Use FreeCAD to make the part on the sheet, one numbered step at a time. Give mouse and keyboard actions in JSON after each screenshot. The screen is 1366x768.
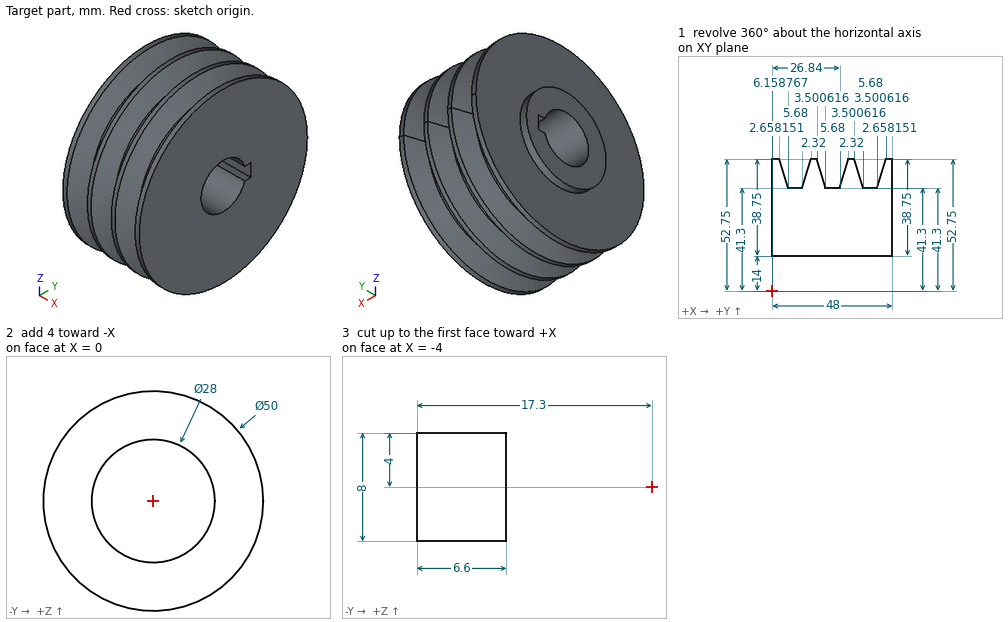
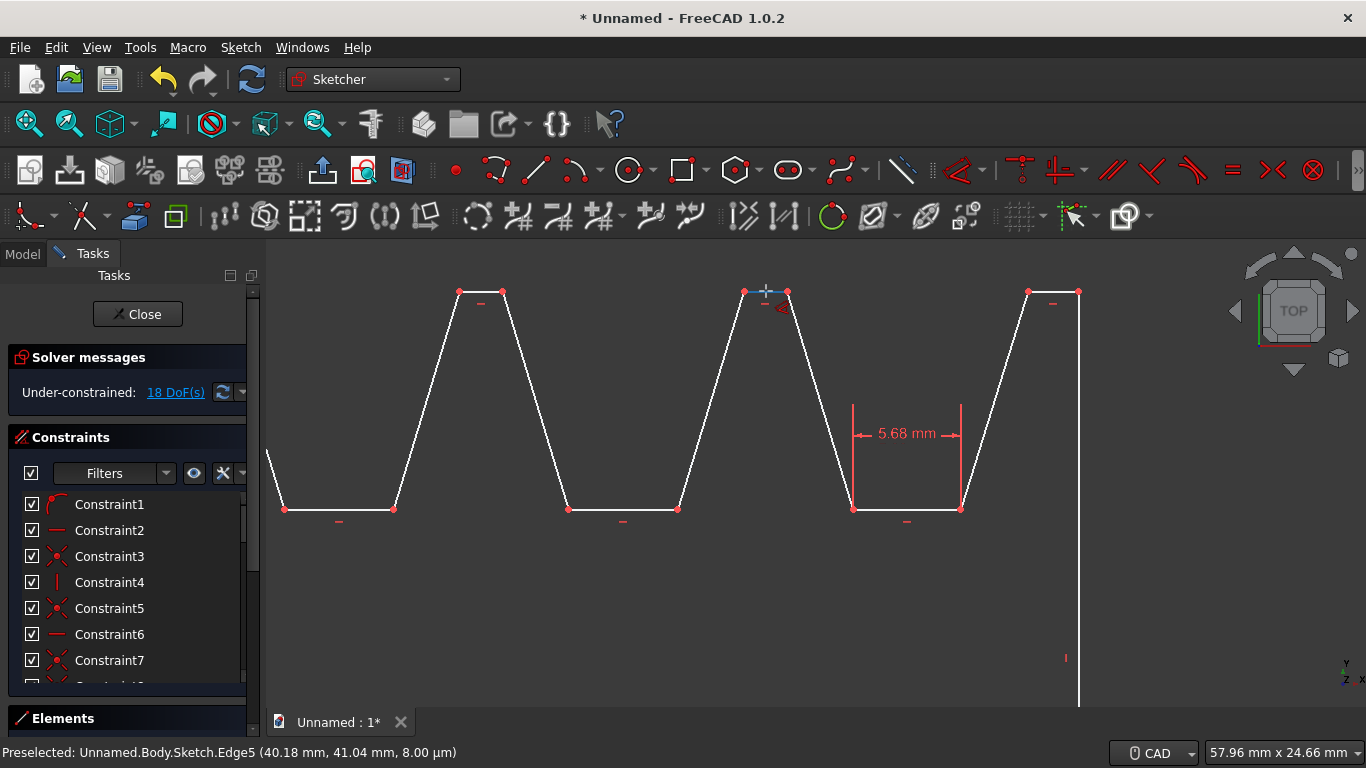
{"action": "left_click", "coordinate": [766, 292]}
{"action": "left_click", "coordinate": [766, 326]}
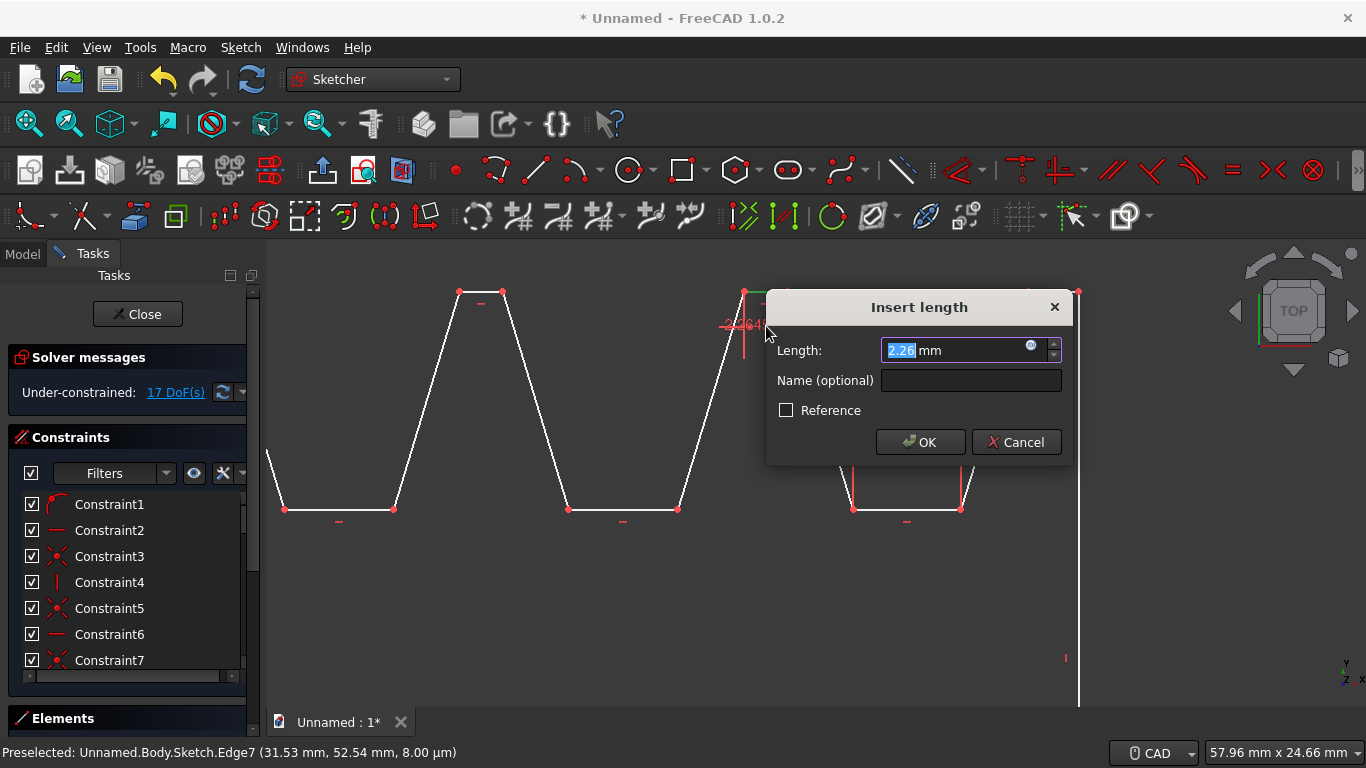
{"action": "type", "text": "2.32"}
{"action": "key", "text": "Return"}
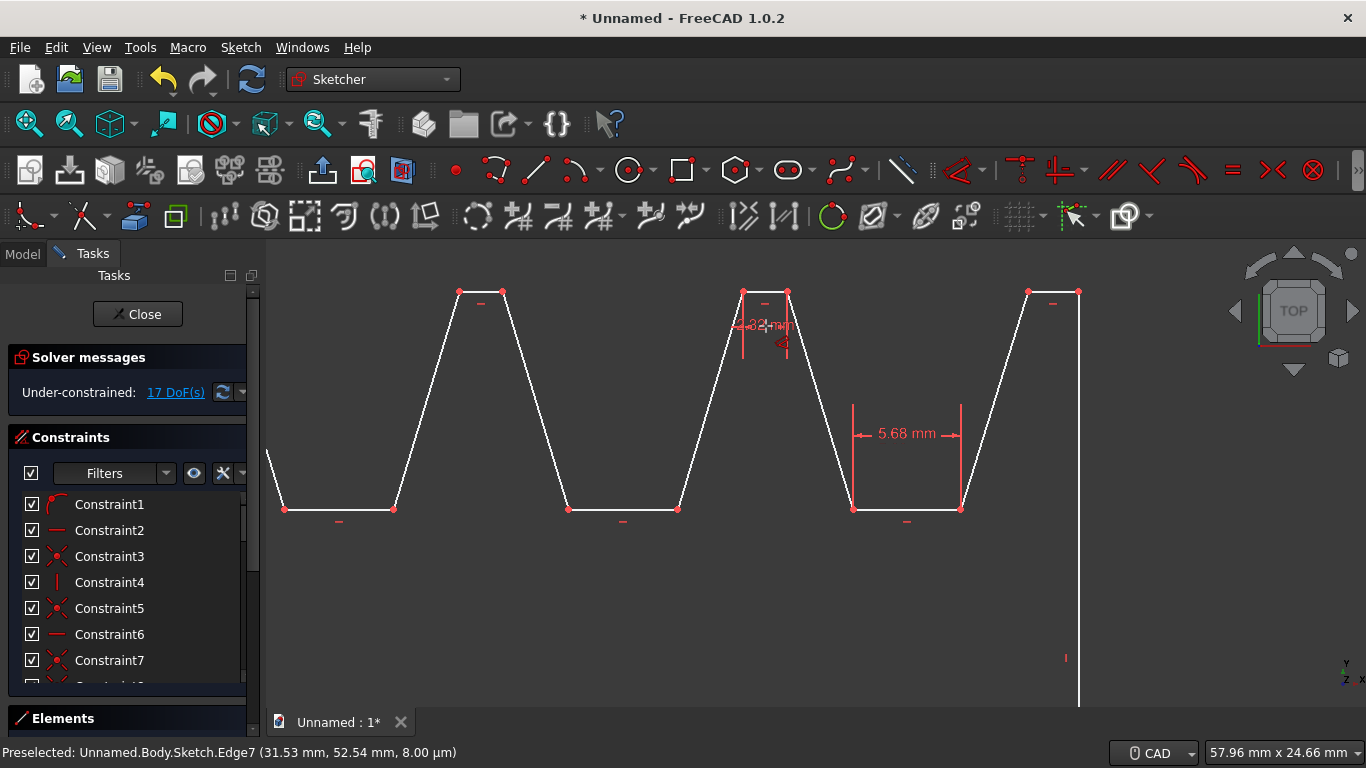
{"action": "left_click", "coordinate": [645, 510]}
{"action": "left_click", "coordinate": [623, 476]}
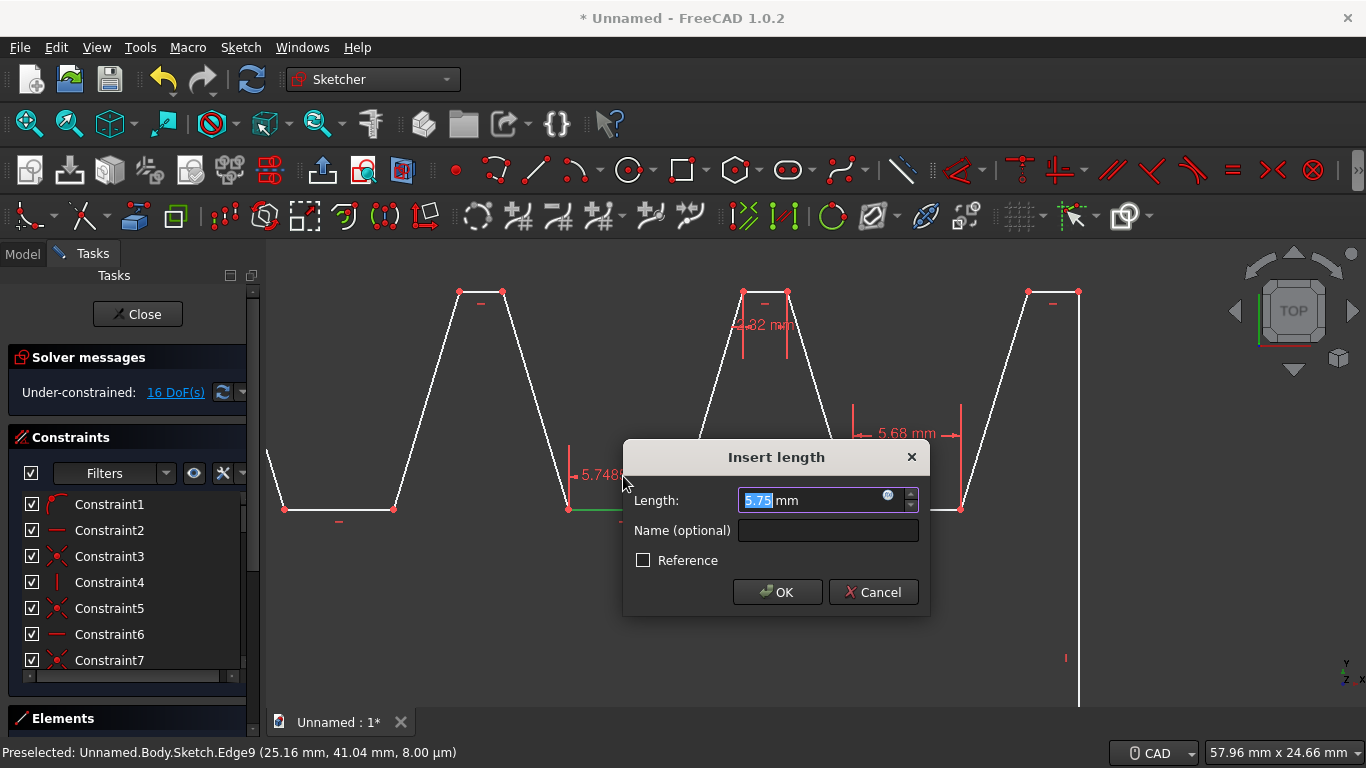
{"action": "type", "text": "5.68"}
{"action": "key", "text": "Return"}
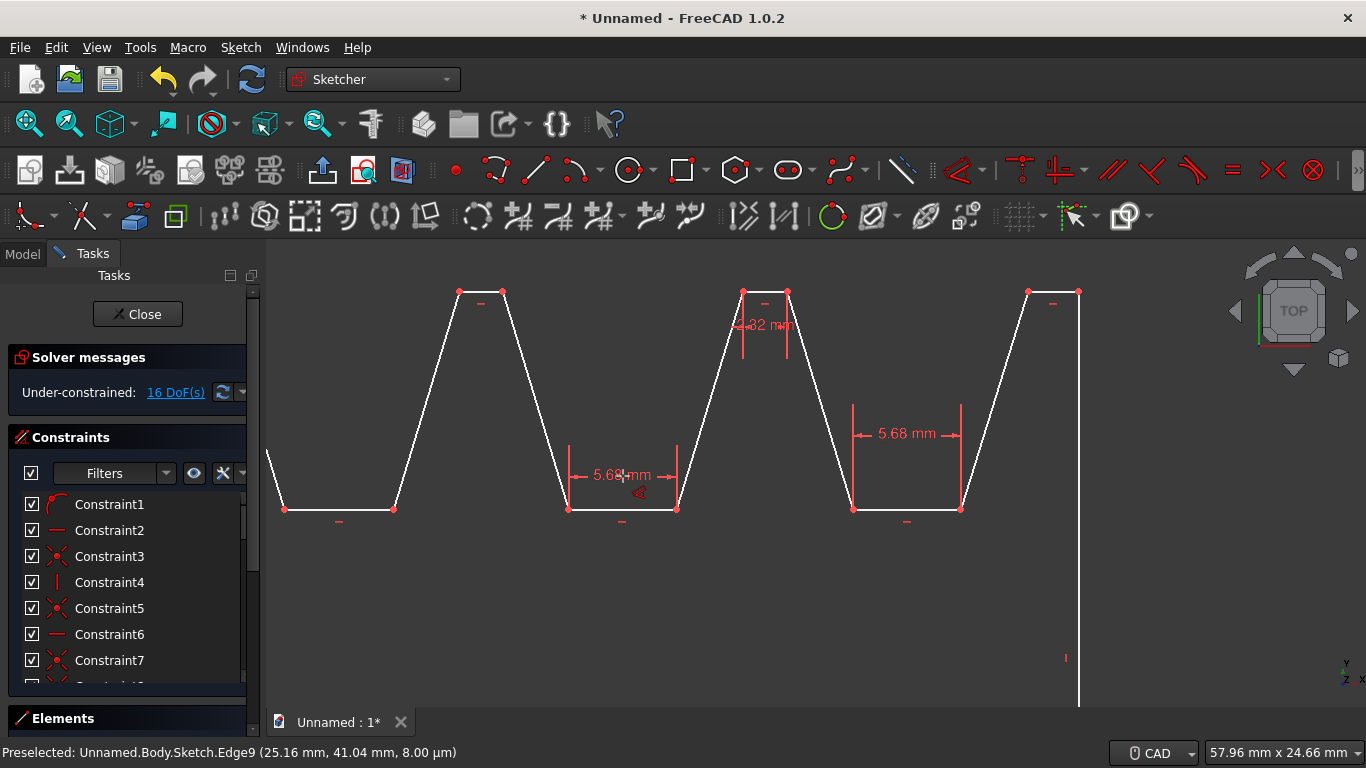
{"action": "left_click", "coordinate": [490, 292]}
{"action": "left_click", "coordinate": [481, 326]}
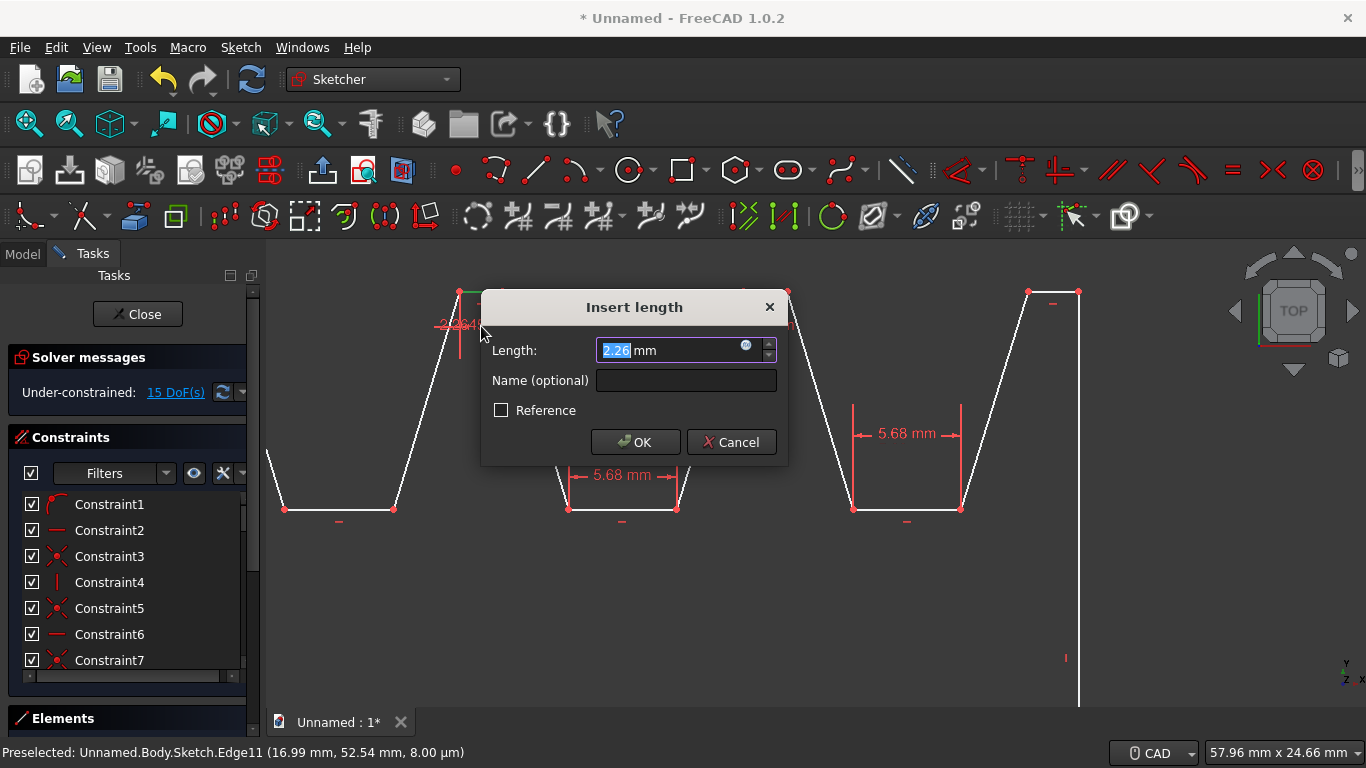
{"action": "type", "text": "2.32"}
{"action": "key", "text": "Return"}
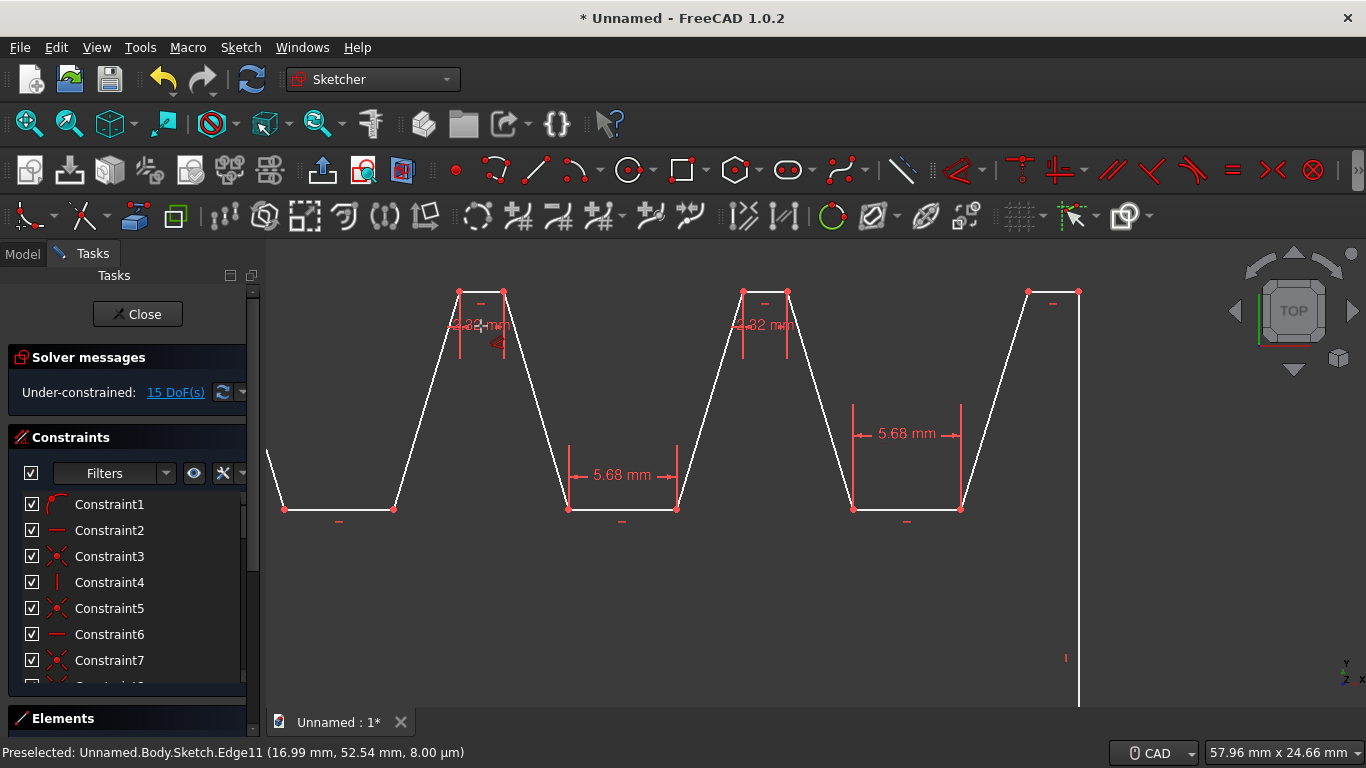
{"action": "left_click", "coordinate": [361, 510]}
{"action": "left_click", "coordinate": [344, 476]}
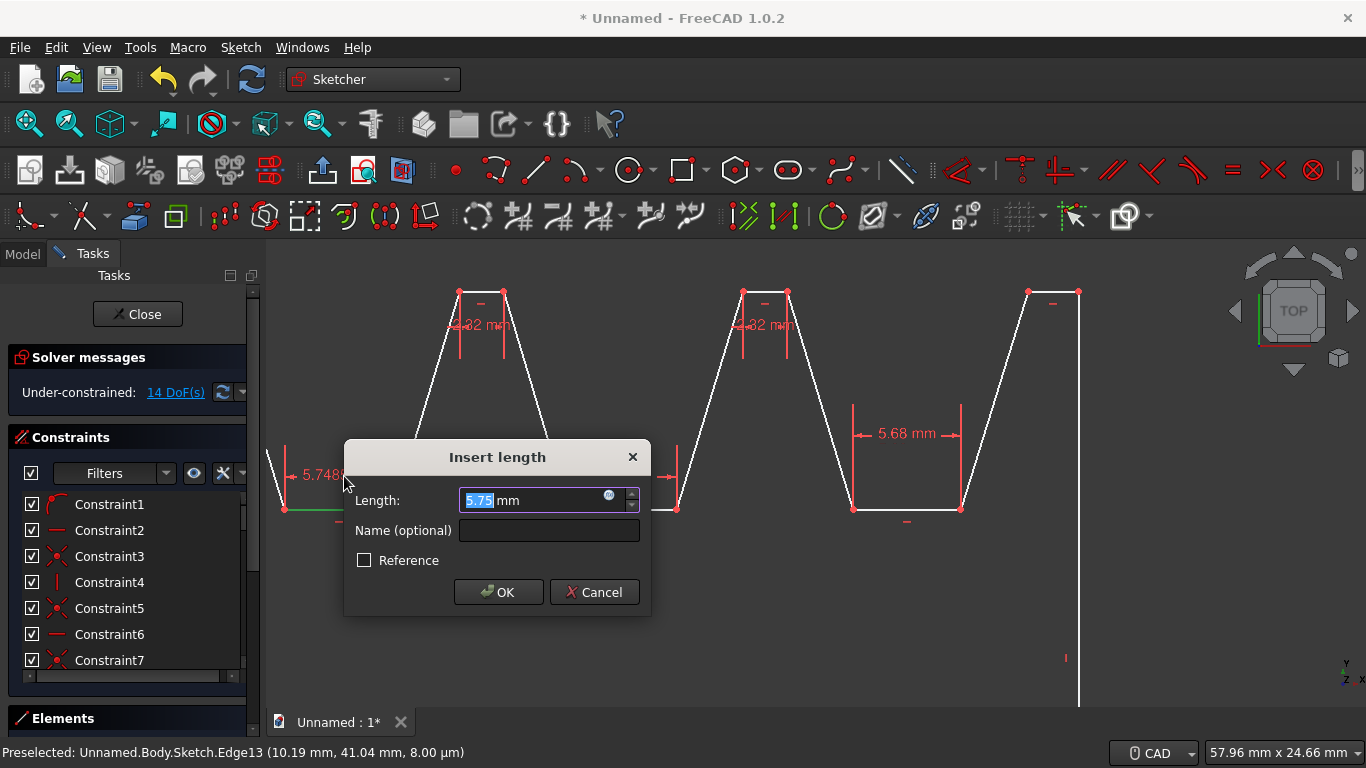
{"action": "type", "text": "5.68"}
{"action": "key", "text": "Return"}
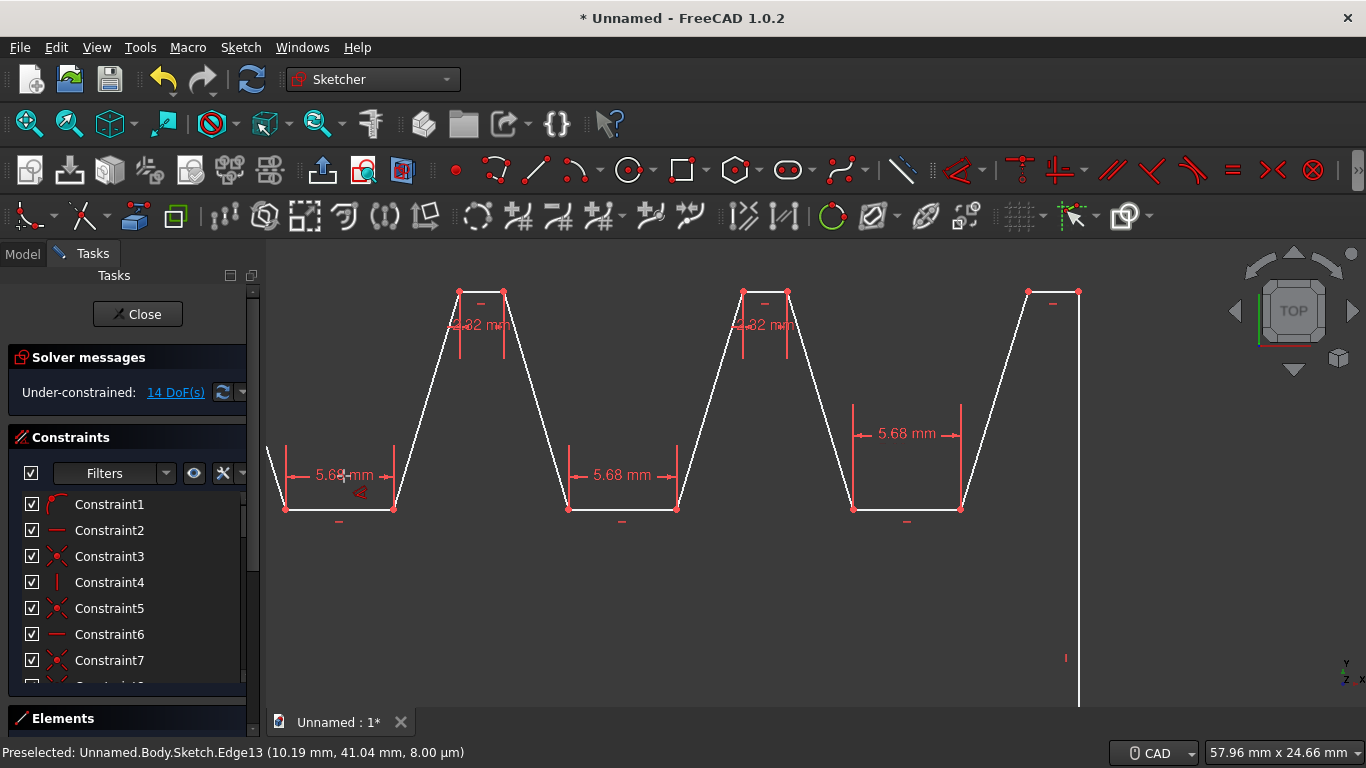
{"action": "left_click", "coordinate": [1079, 511]}
{"action": "left_click", "coordinate": [1113, 485]}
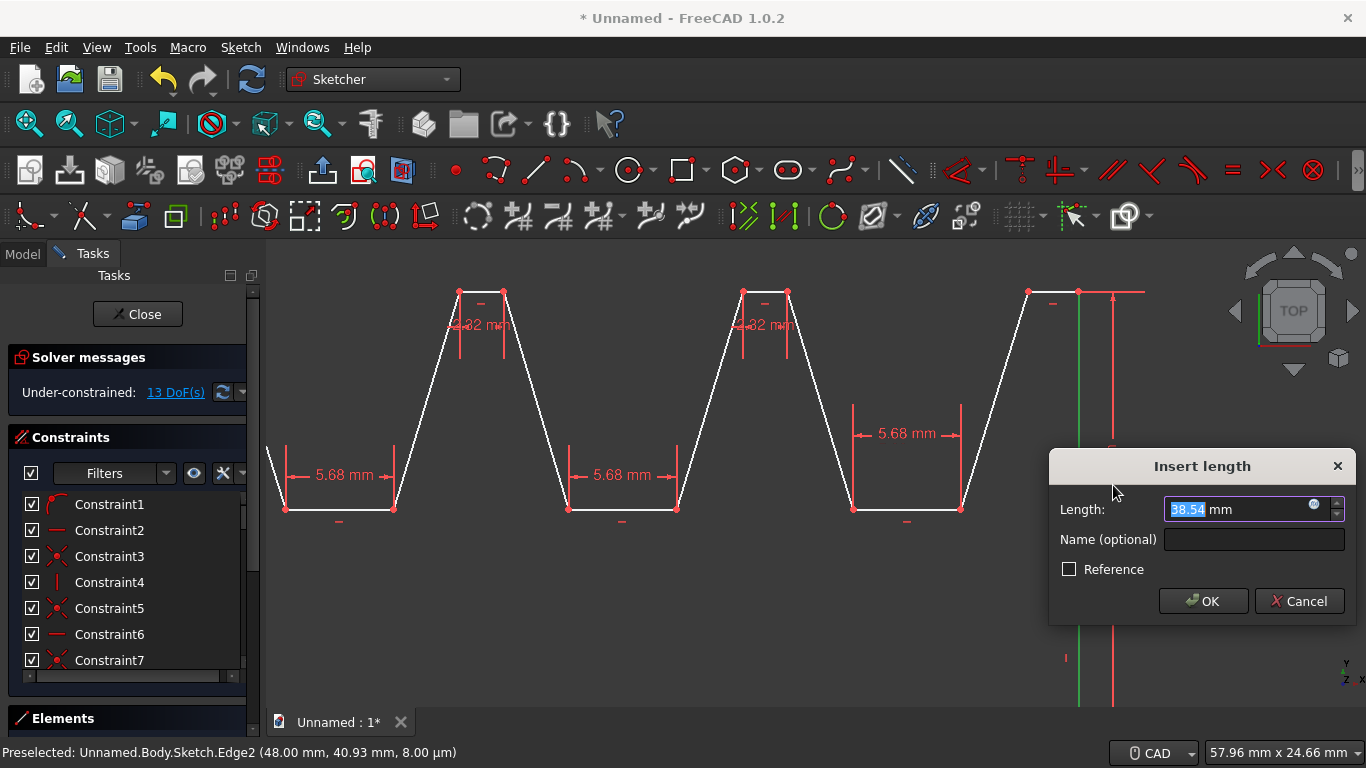
{"action": "type", "text": "38.75"}
{"action": "key", "text": "Return"}